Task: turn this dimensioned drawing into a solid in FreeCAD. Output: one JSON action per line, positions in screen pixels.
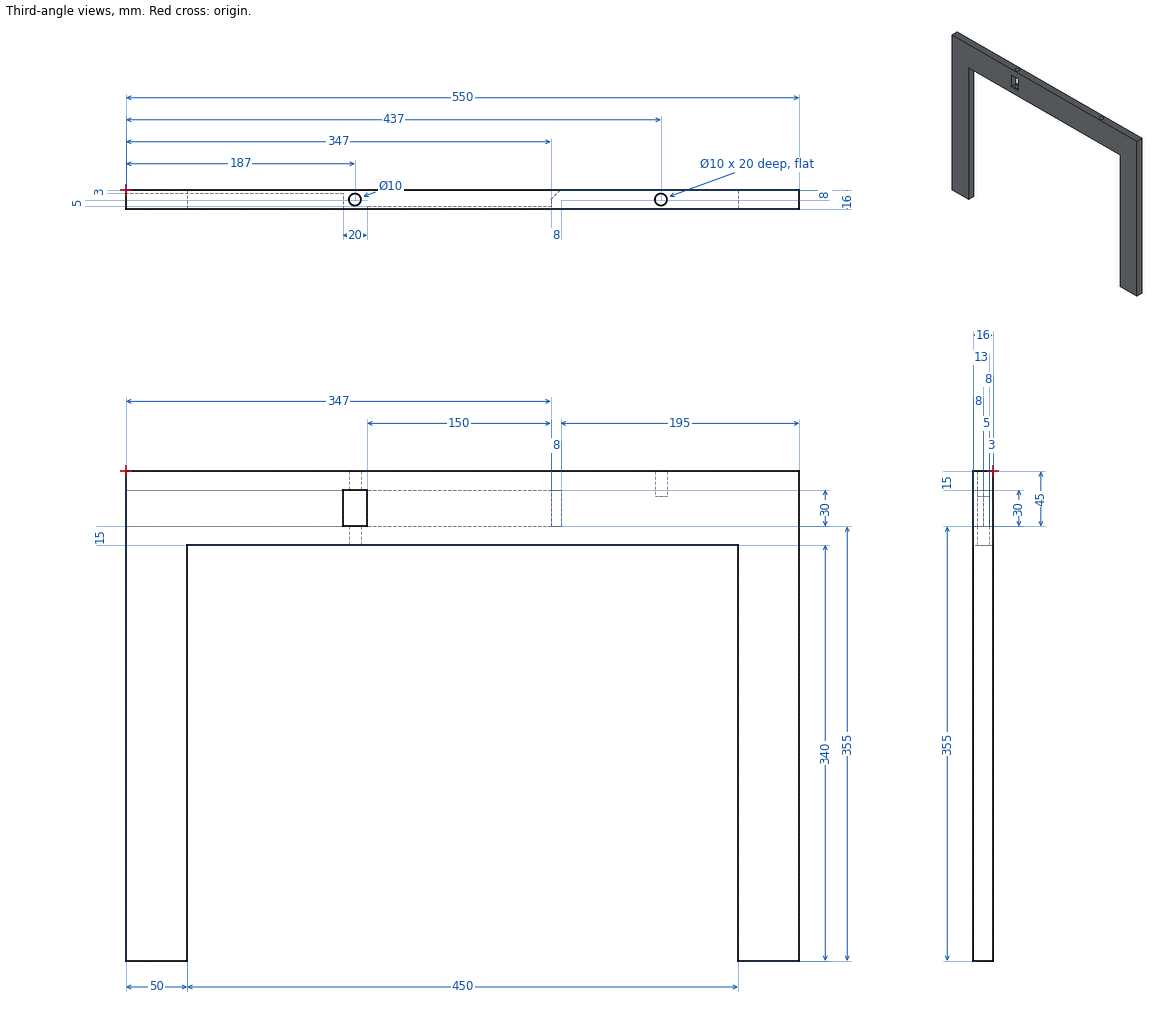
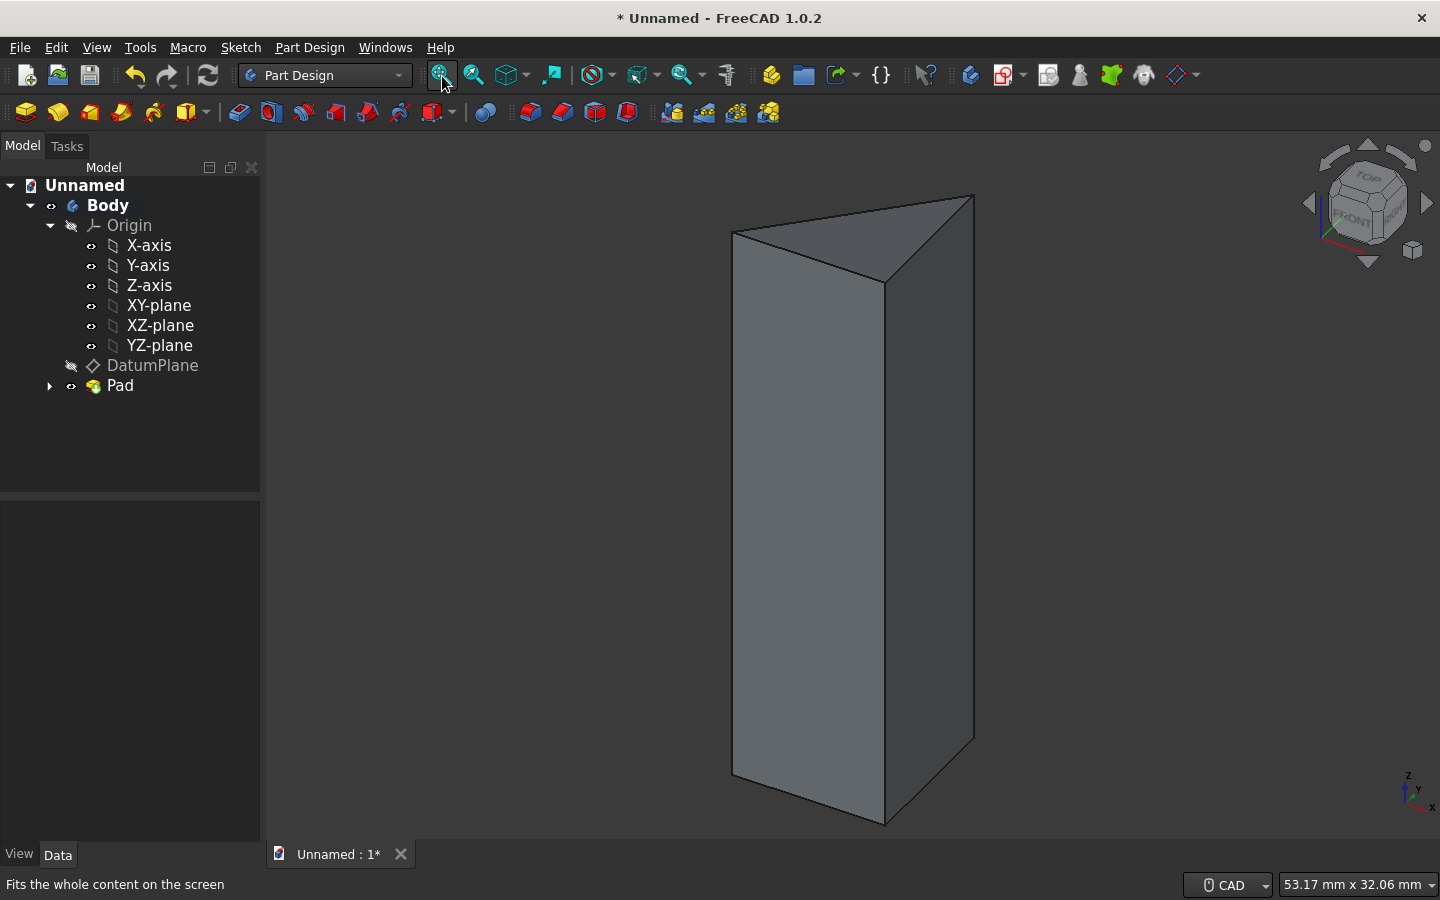
{"action": "left_click", "coordinate": [809, 373]}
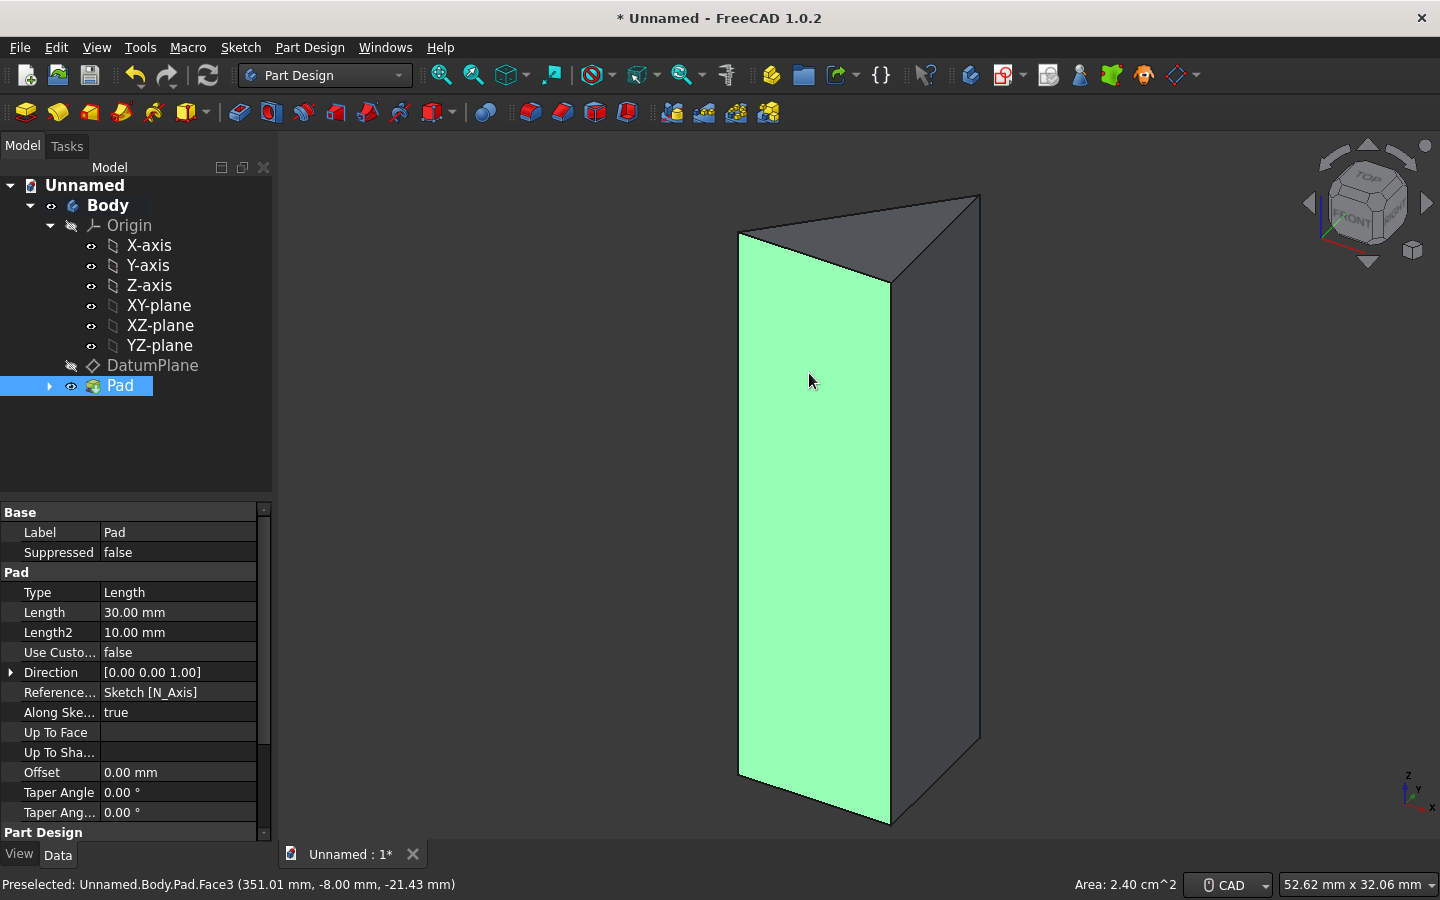
{"action": "left_click", "coordinate": [1004, 76]}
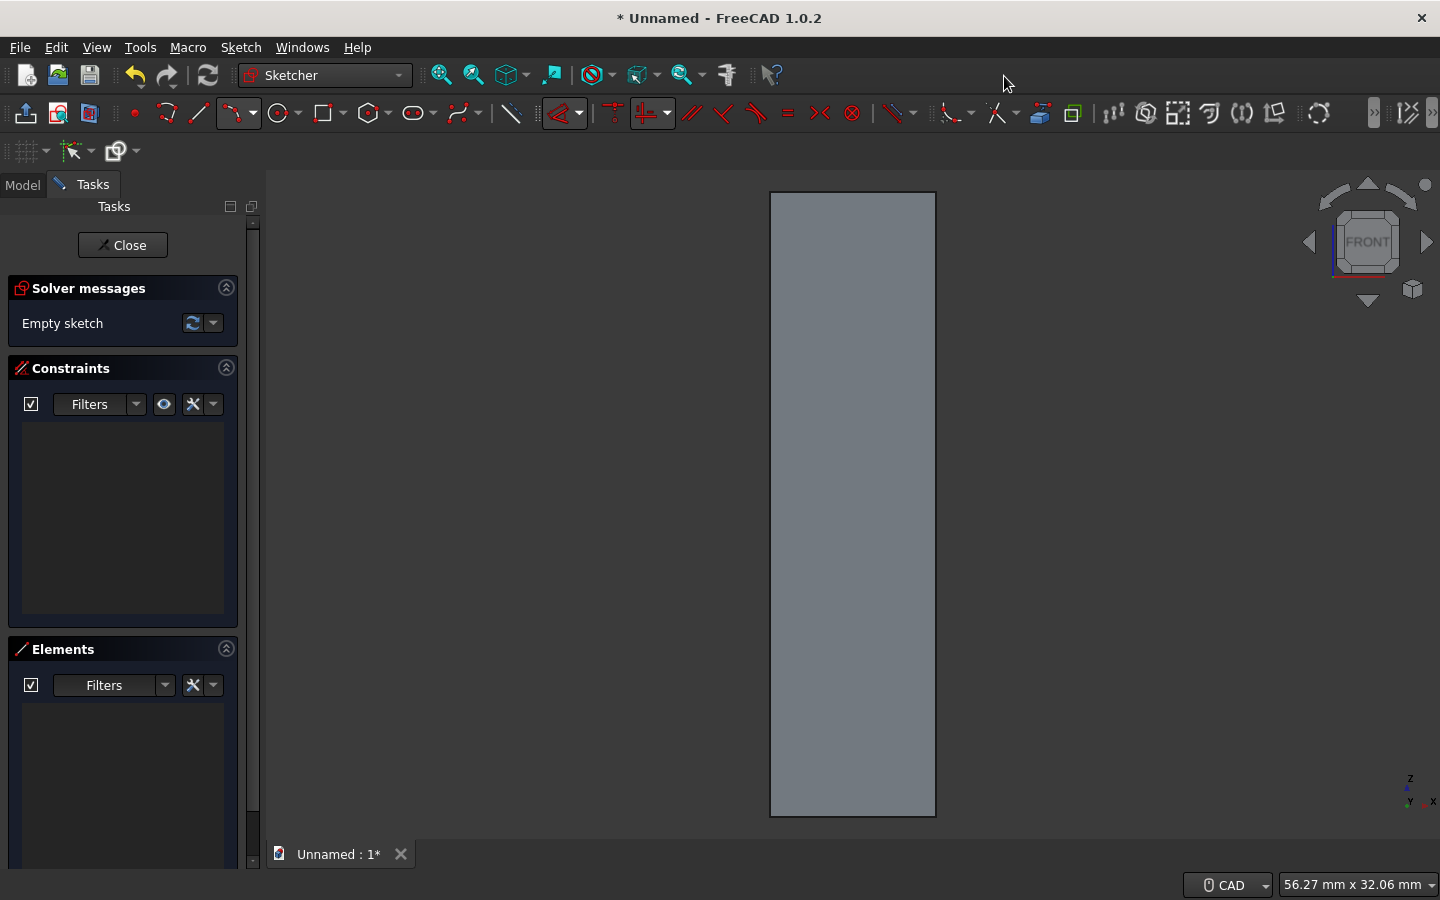
{"action": "scroll", "coordinate": [645, 504], "scroll_direction": "down", "scroll_amount": 2}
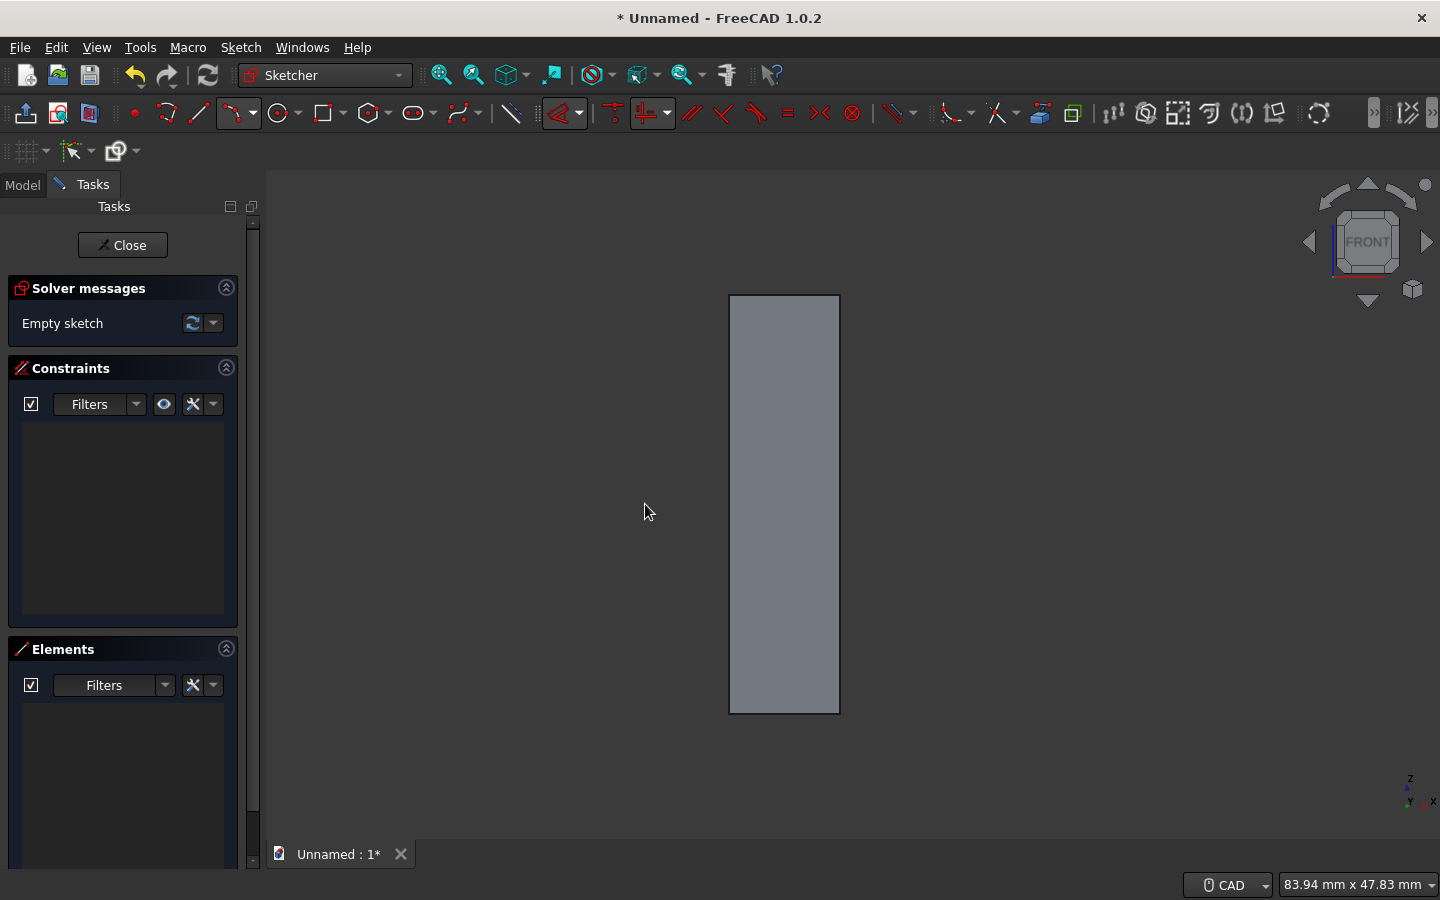
{"action": "left_click", "coordinate": [324, 114]}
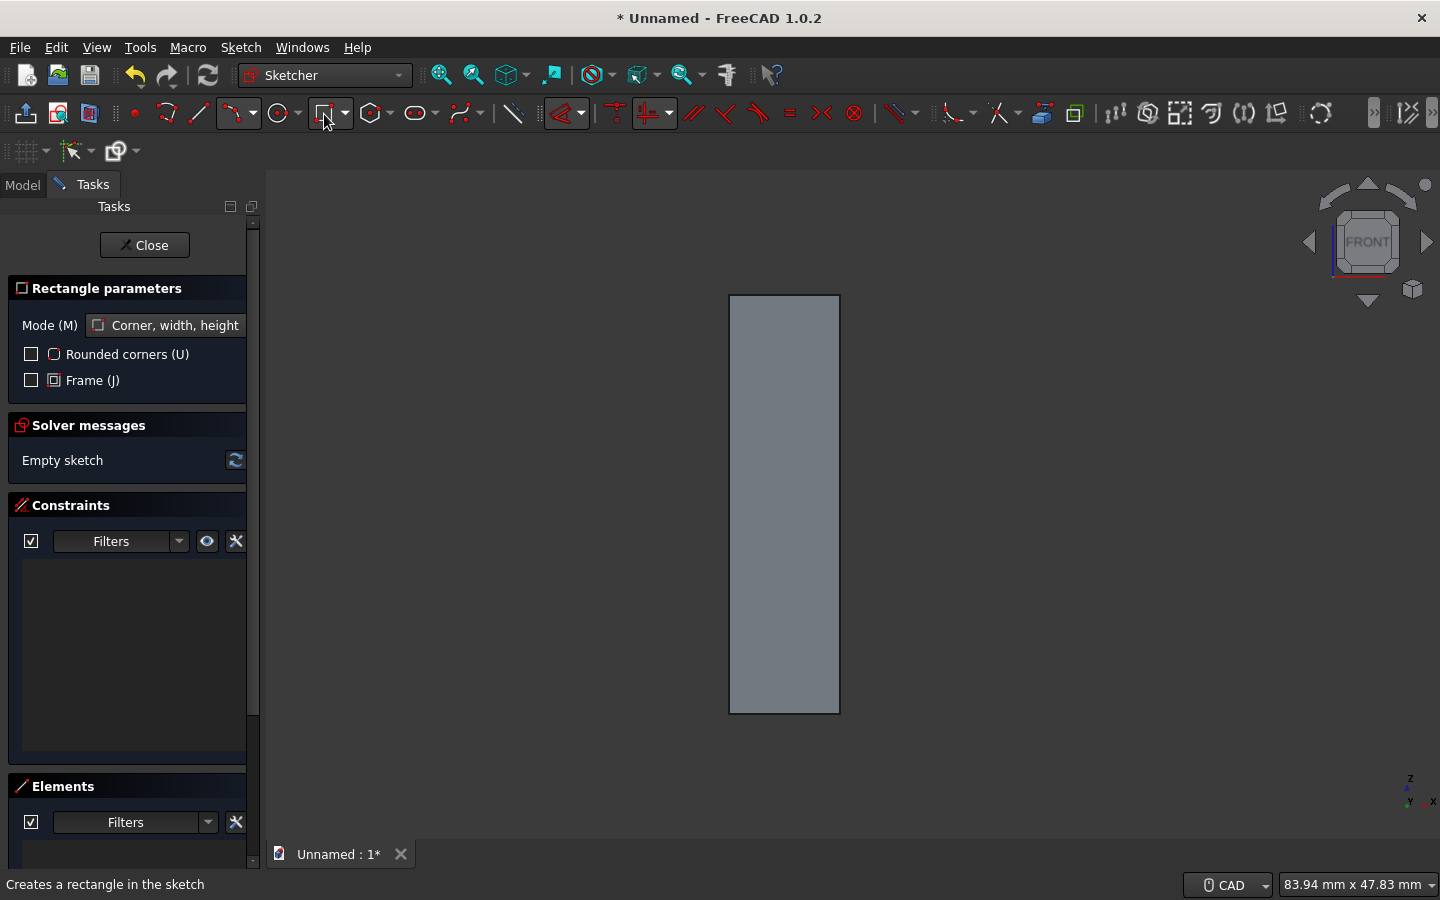
{"action": "left_click", "coordinate": [729, 295]}
{"action": "left_click", "coordinate": [840, 714]}
{"action": "key", "text": "Escape"}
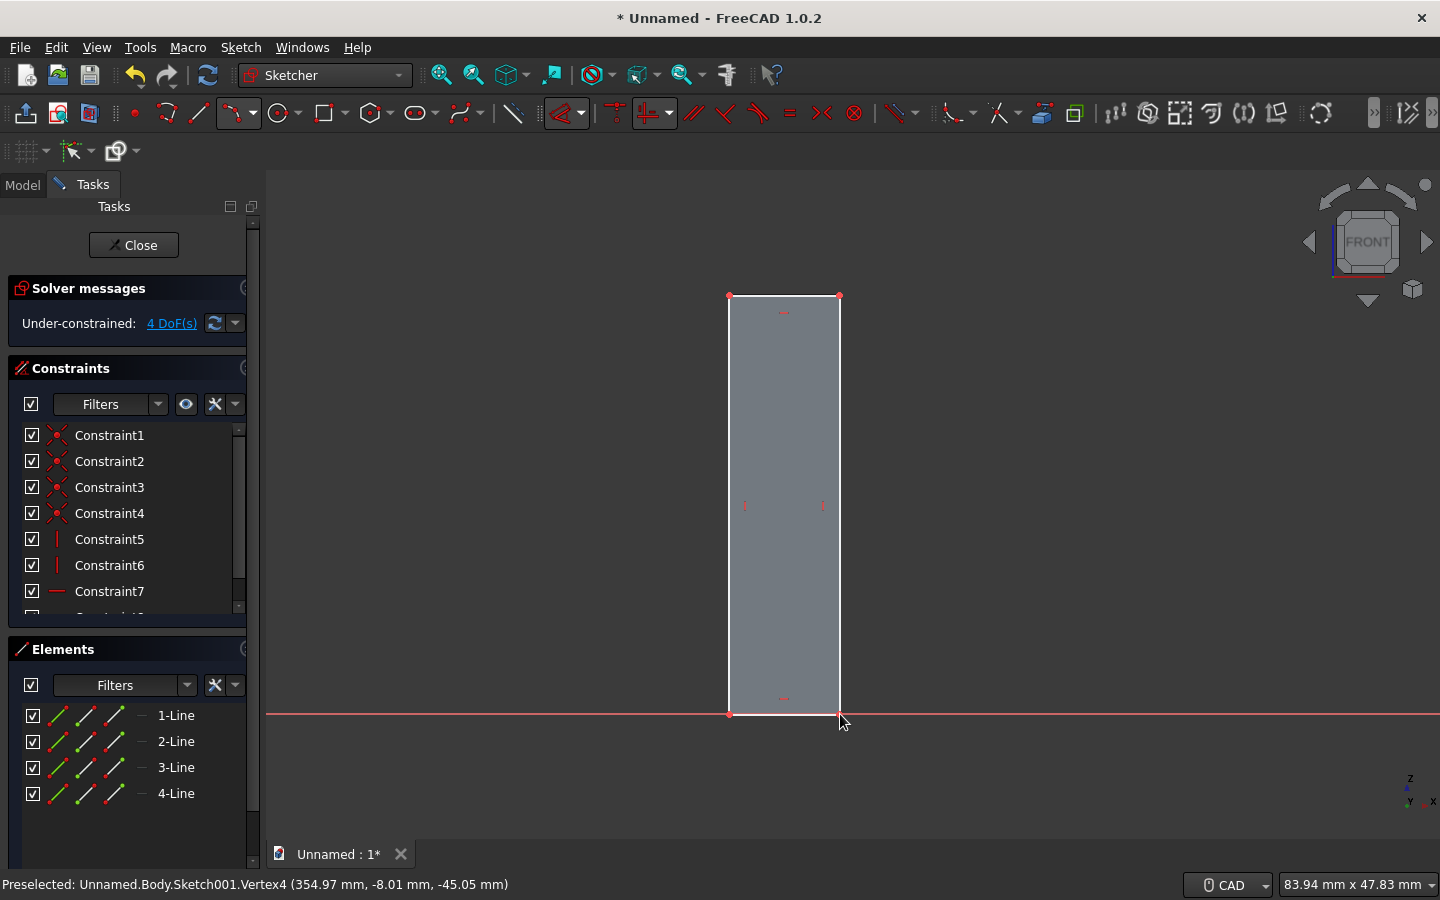
{"action": "left_click", "coordinate": [729, 715]}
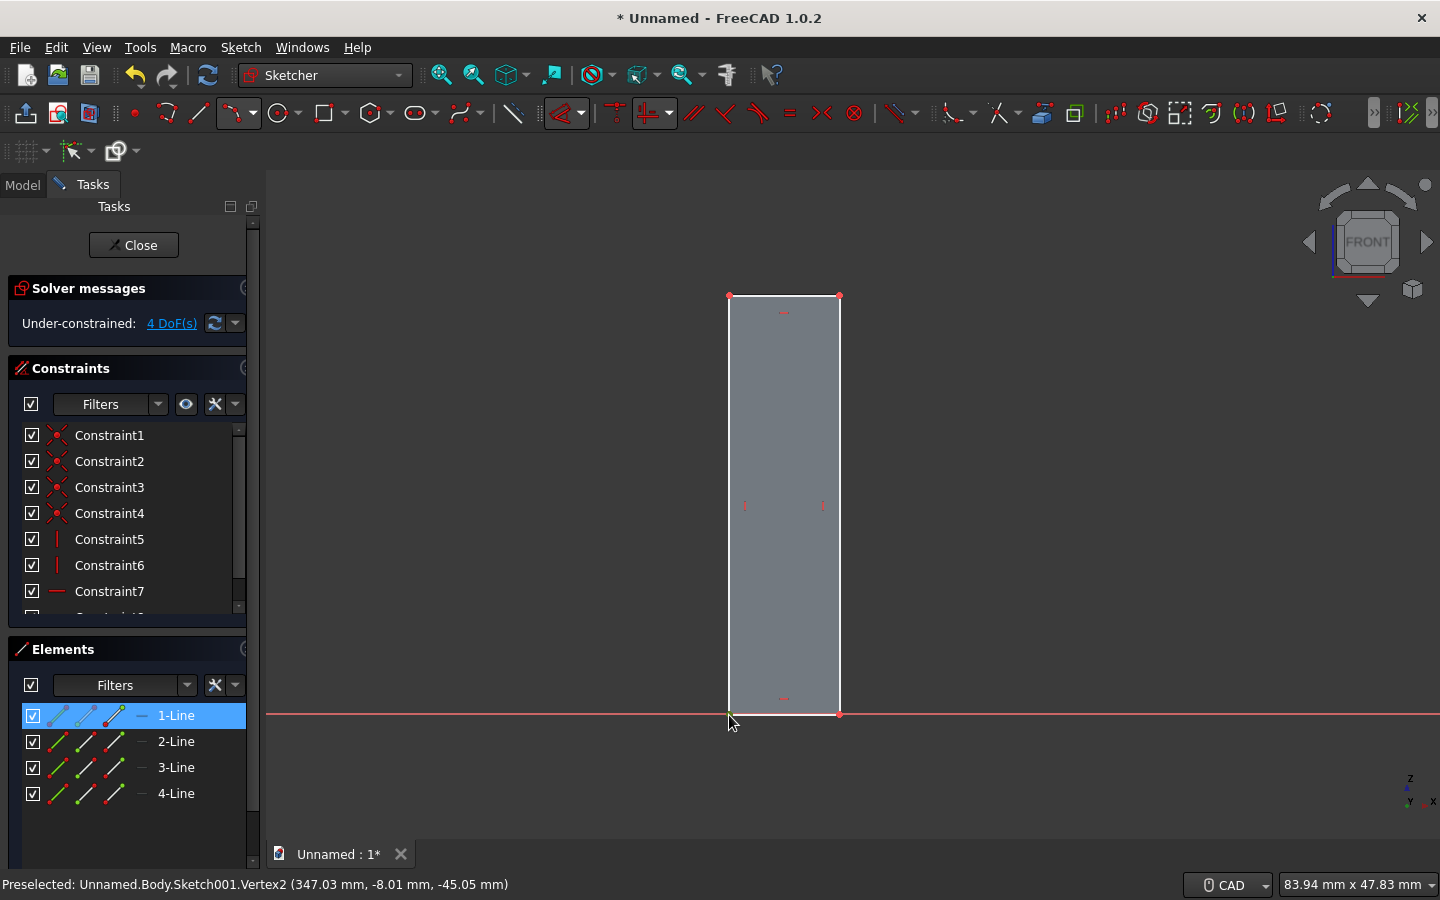
{"action": "left_click", "coordinate": [364, 714]}